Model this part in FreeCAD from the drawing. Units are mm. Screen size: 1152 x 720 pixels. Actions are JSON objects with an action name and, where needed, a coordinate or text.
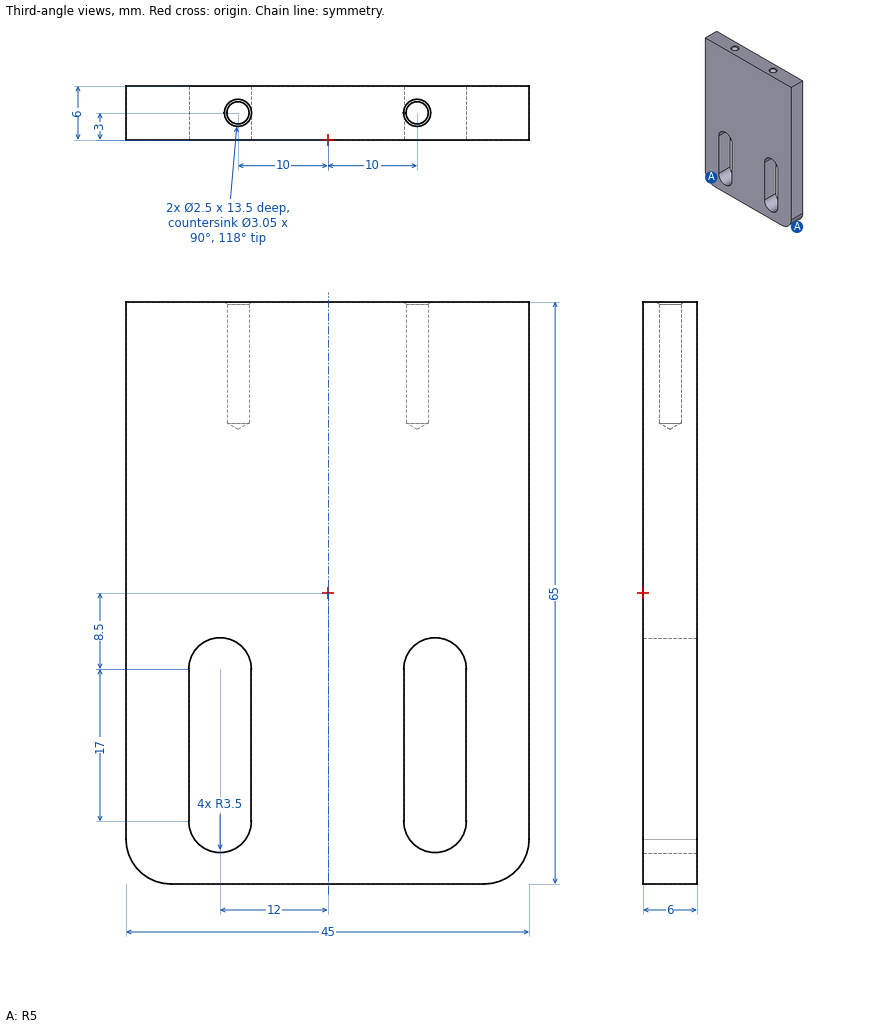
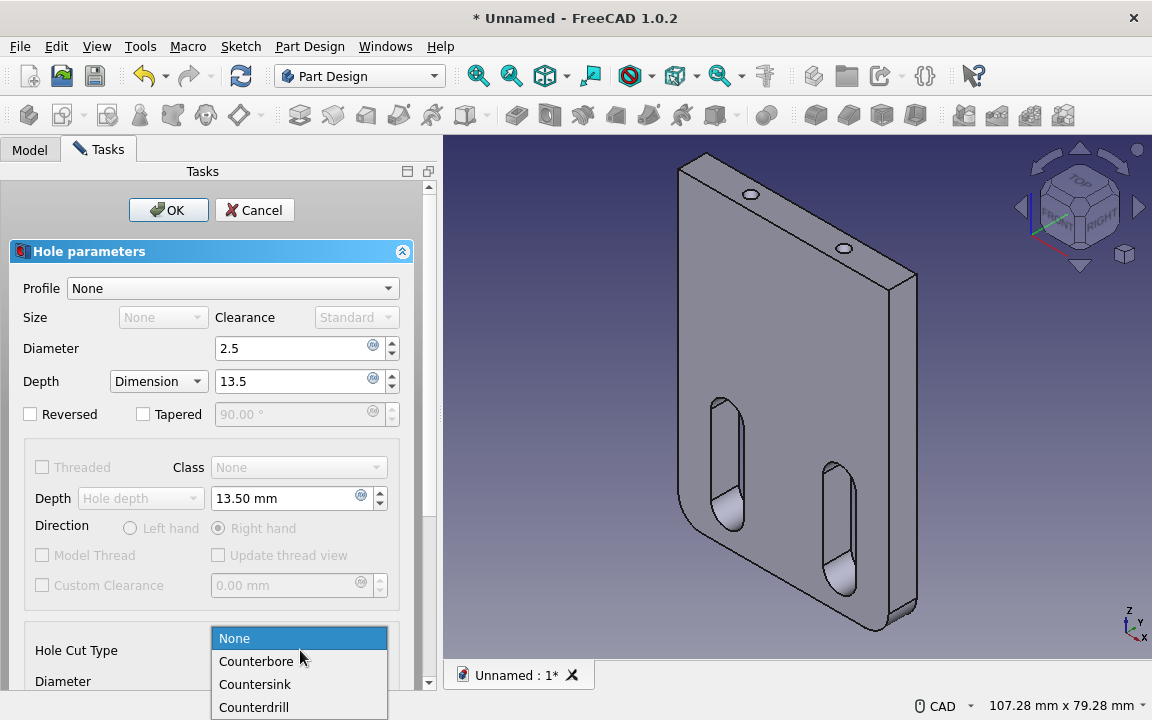
{"action": "left_click", "coordinate": [298, 684]}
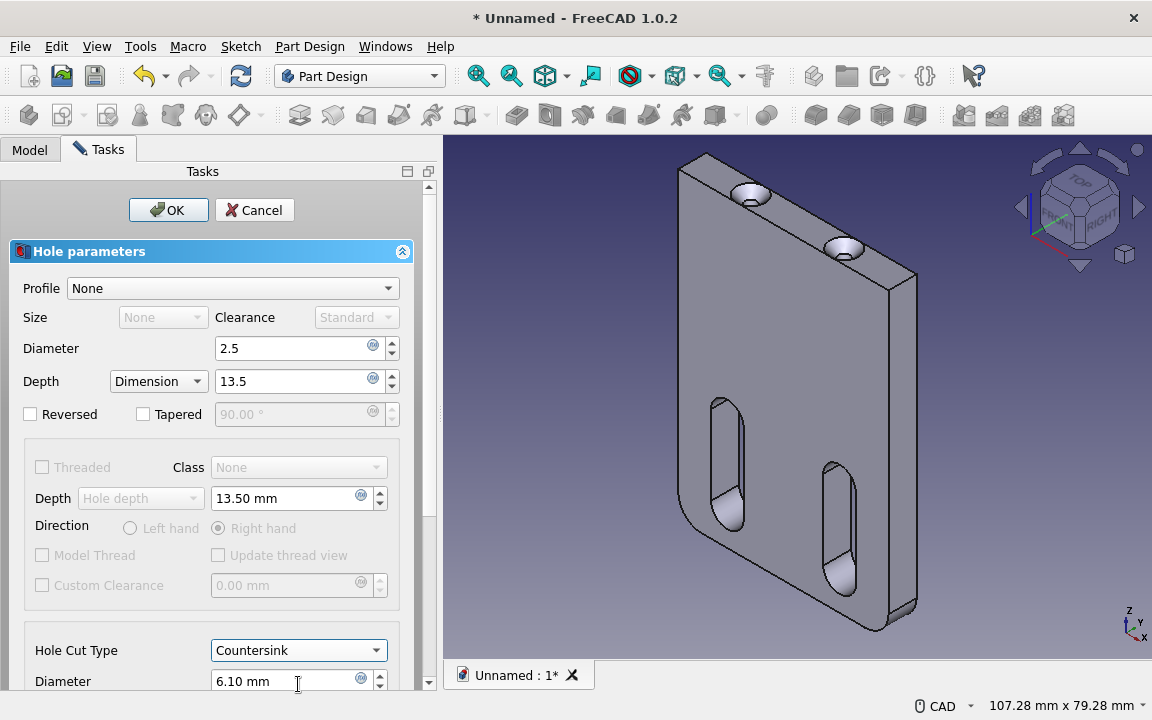
{"action": "scroll", "coordinate": [429, 436], "scroll_direction": "down", "scroll_amount": 2}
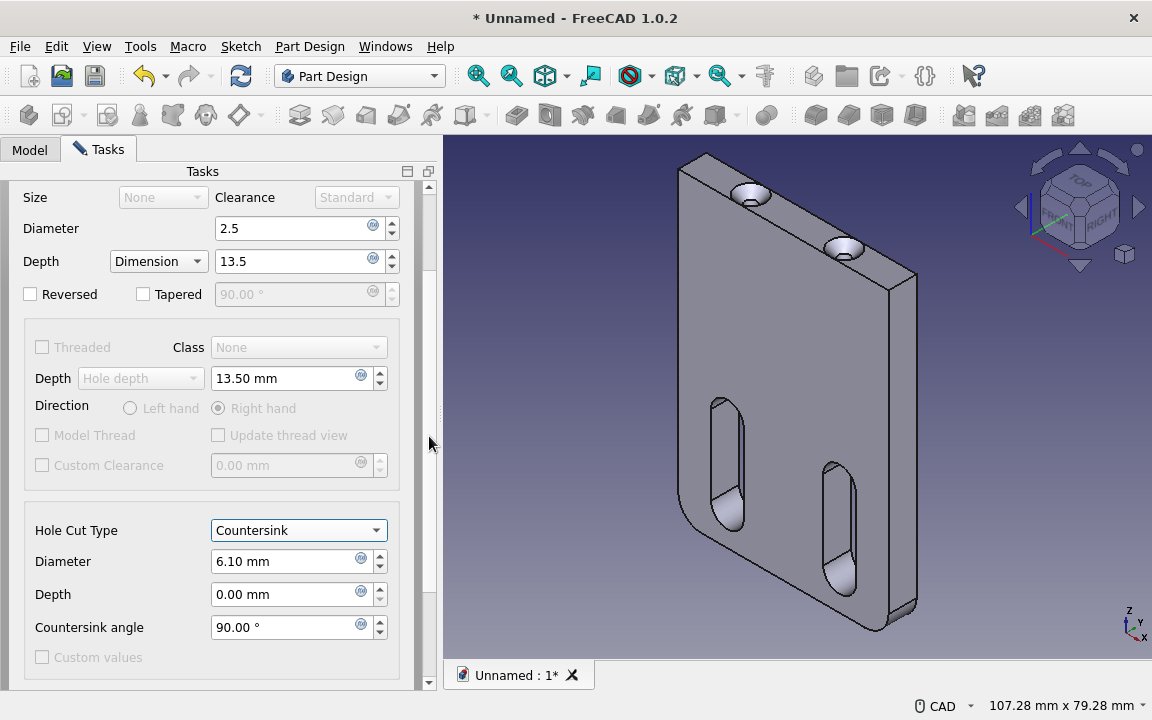
{"action": "triple_click", "coordinate": [292, 562]}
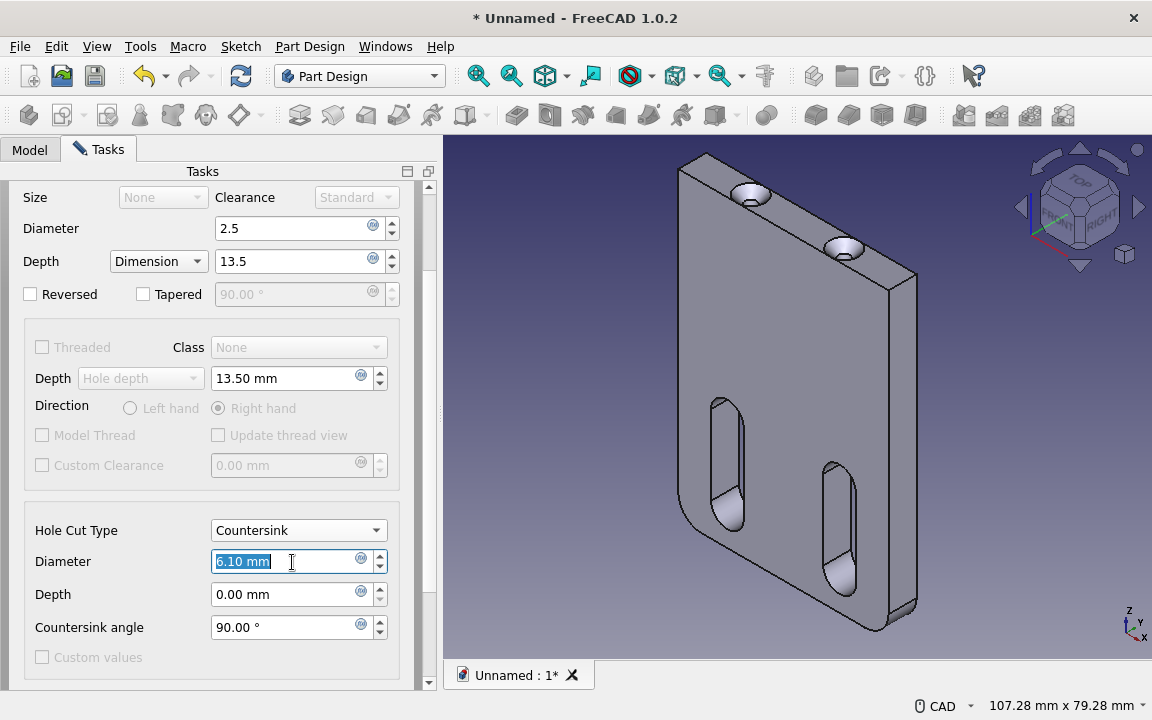
{"action": "type", "text": "3.05"}
{"action": "key", "text": "Tab"}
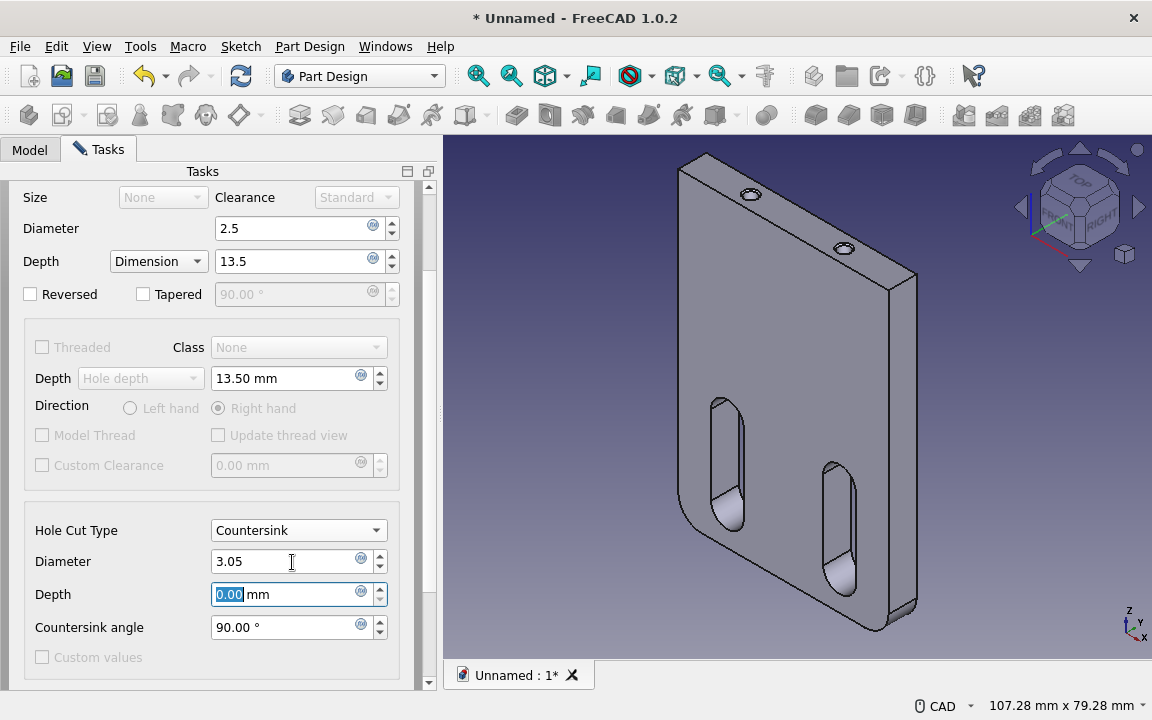
{"action": "scroll", "coordinate": [429, 436], "scroll_direction": "up", "scroll_amount": 3}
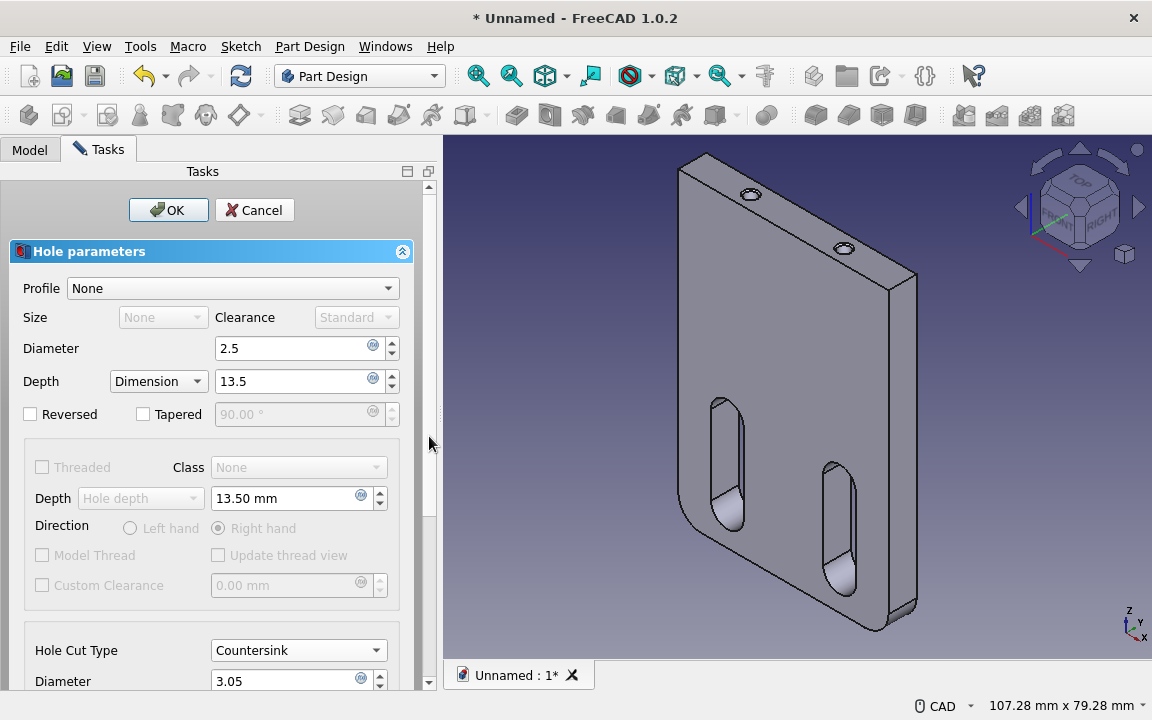
{"action": "left_click", "coordinate": [169, 210]}